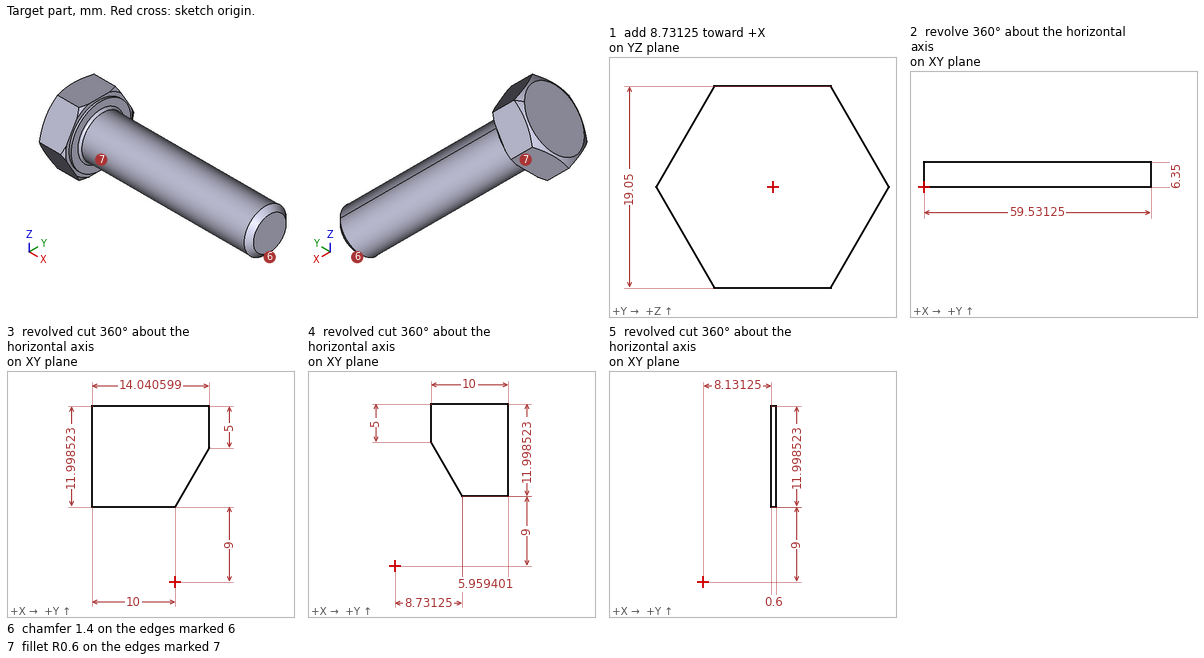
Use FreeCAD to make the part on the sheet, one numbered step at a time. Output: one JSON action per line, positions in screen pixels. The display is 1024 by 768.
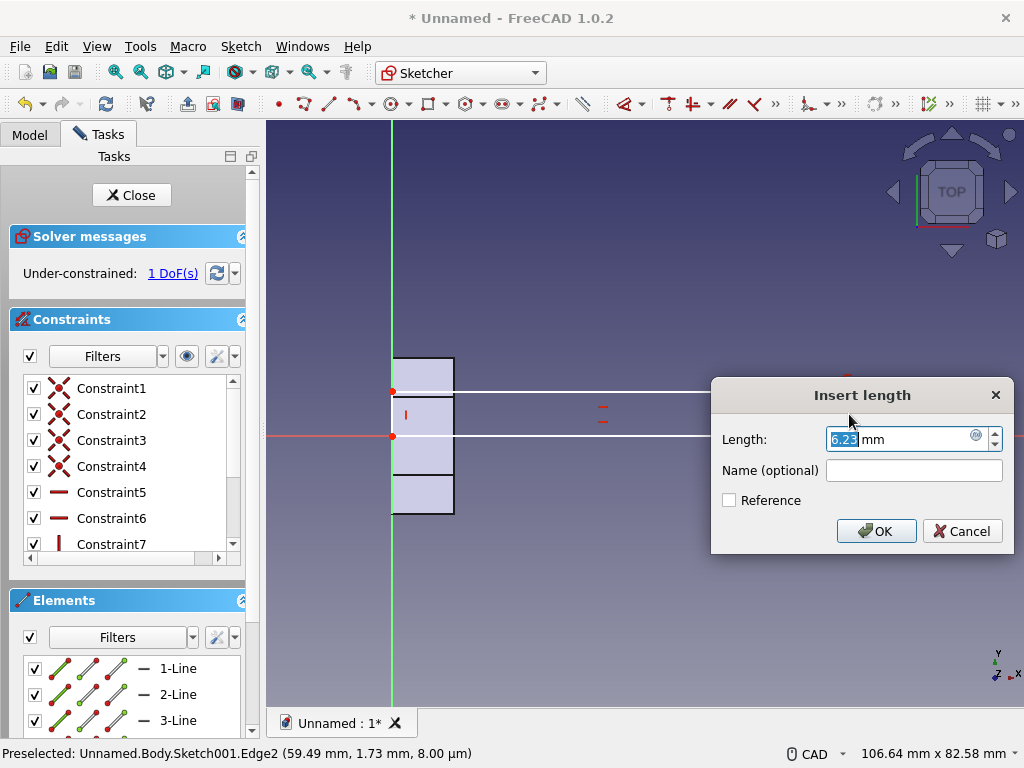
{"action": "type", "text": "6.35"}
{"action": "key", "text": "Return"}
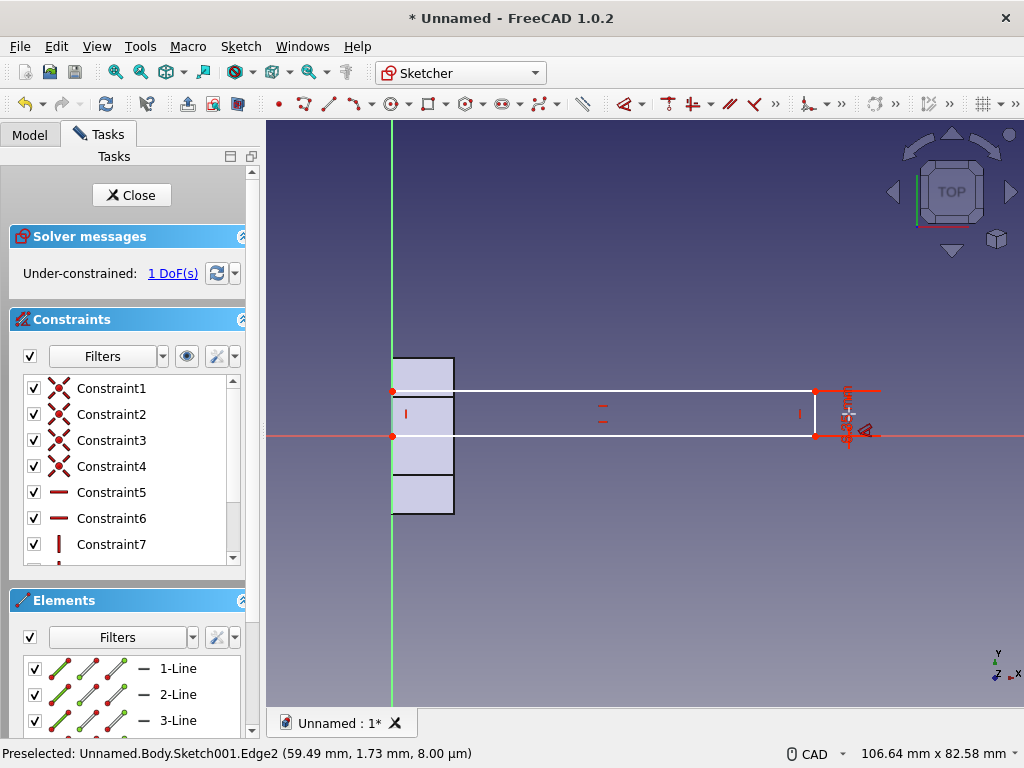
{"action": "left_click", "coordinate": [519, 436]}
{"action": "left_click", "coordinate": [604, 470]}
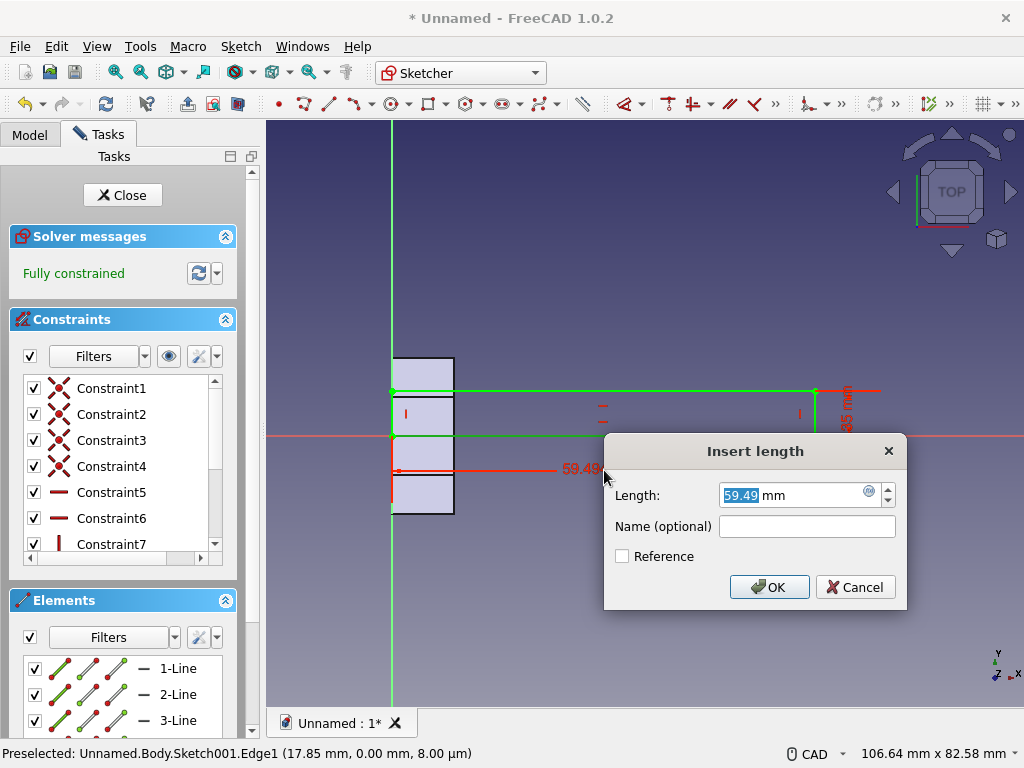
{"action": "type", "text": "59.53125"}
{"action": "key", "text": "Return"}
{"action": "key", "text": "Escape"}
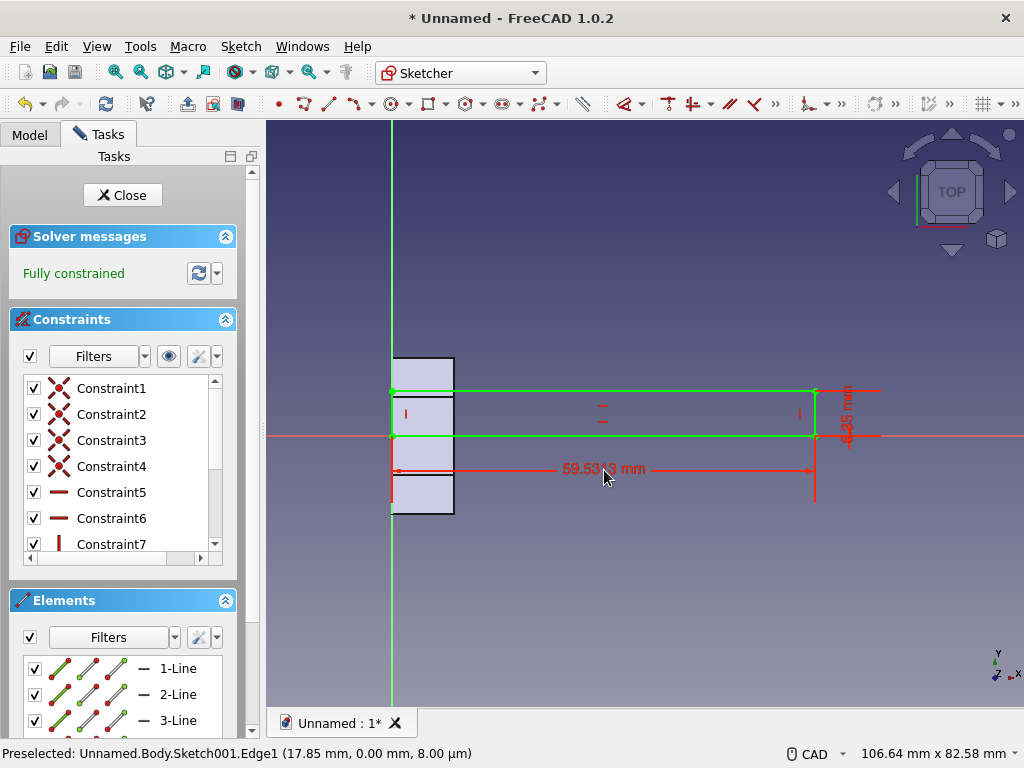
{"action": "left_click", "coordinate": [123, 195]}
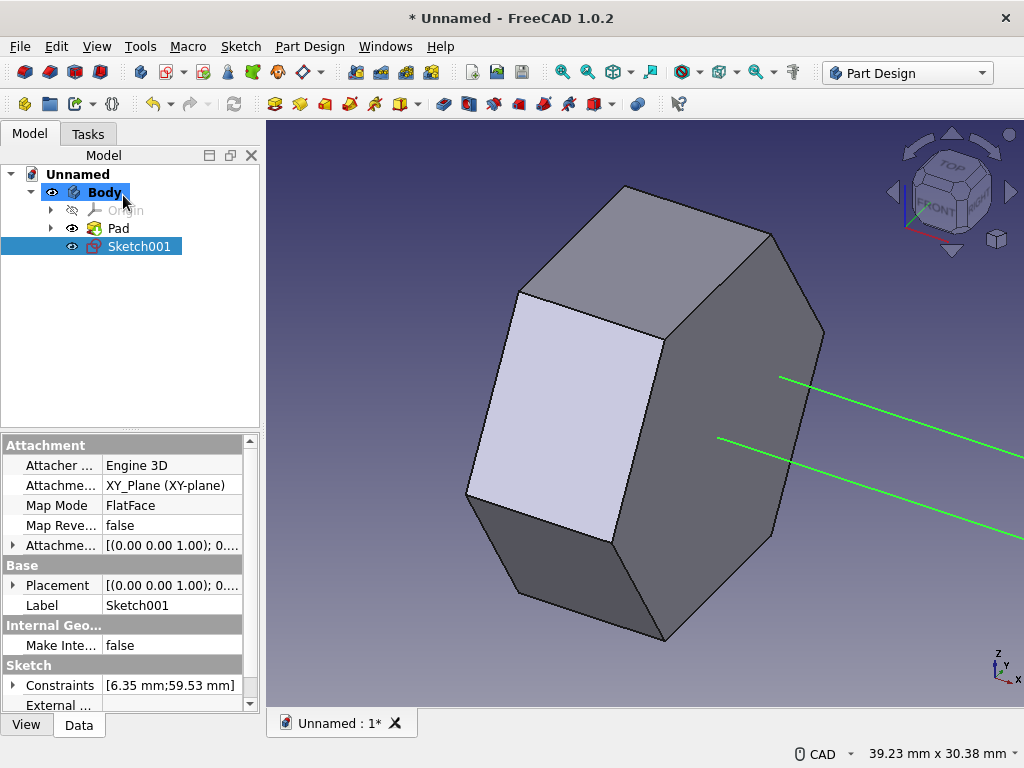
{"action": "left_click", "coordinate": [300, 104]}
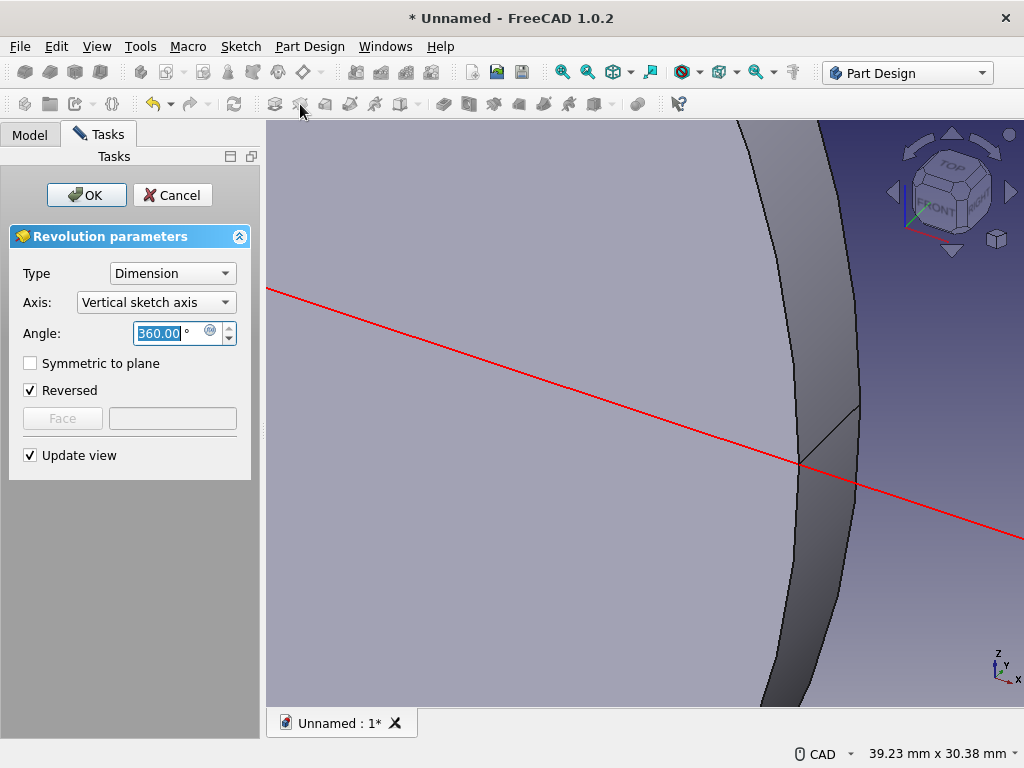
{"action": "left_click", "coordinate": [157, 302]}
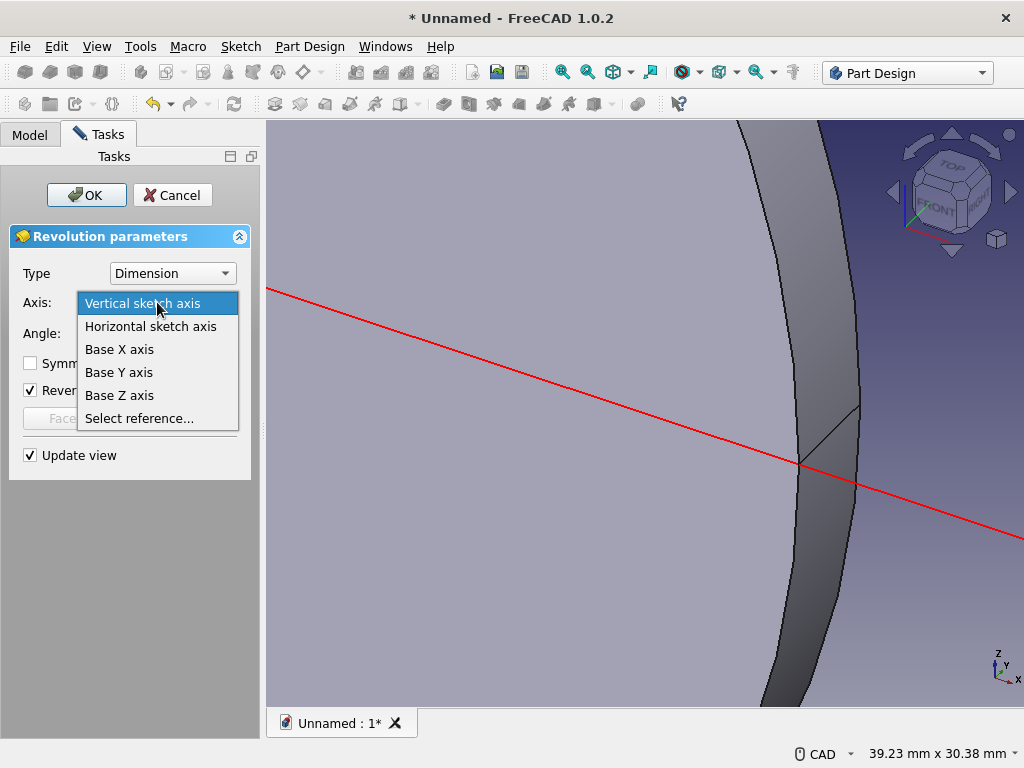
{"action": "left_click", "coordinate": [156, 326]}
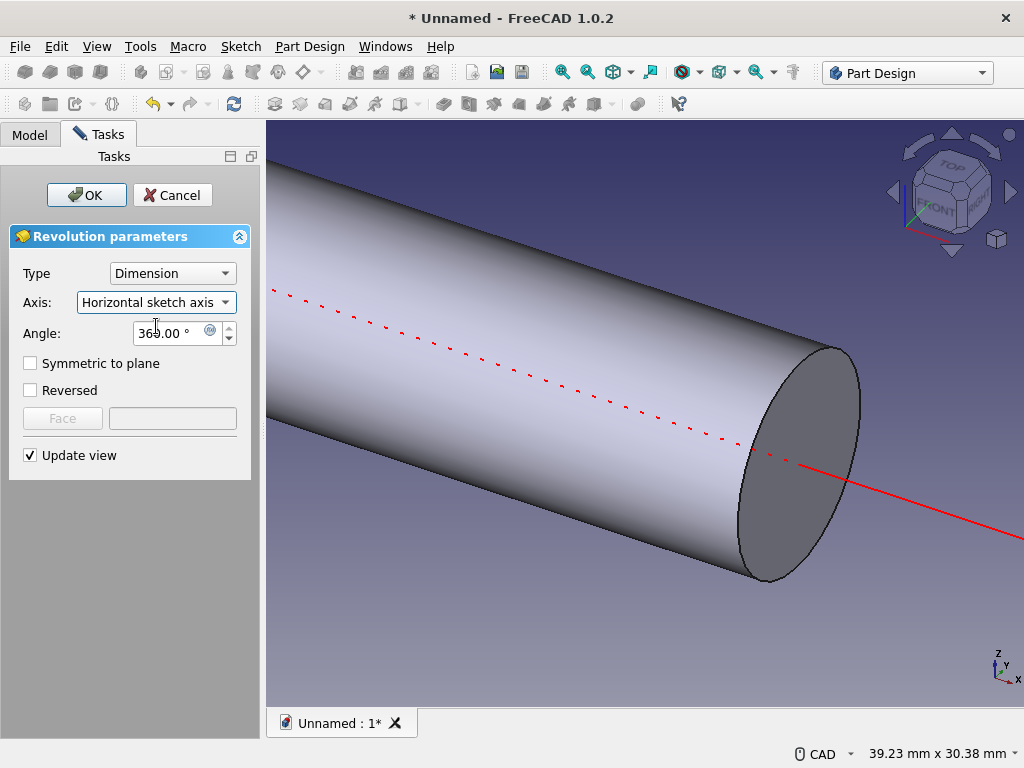
{"action": "left_click", "coordinate": [87, 195]}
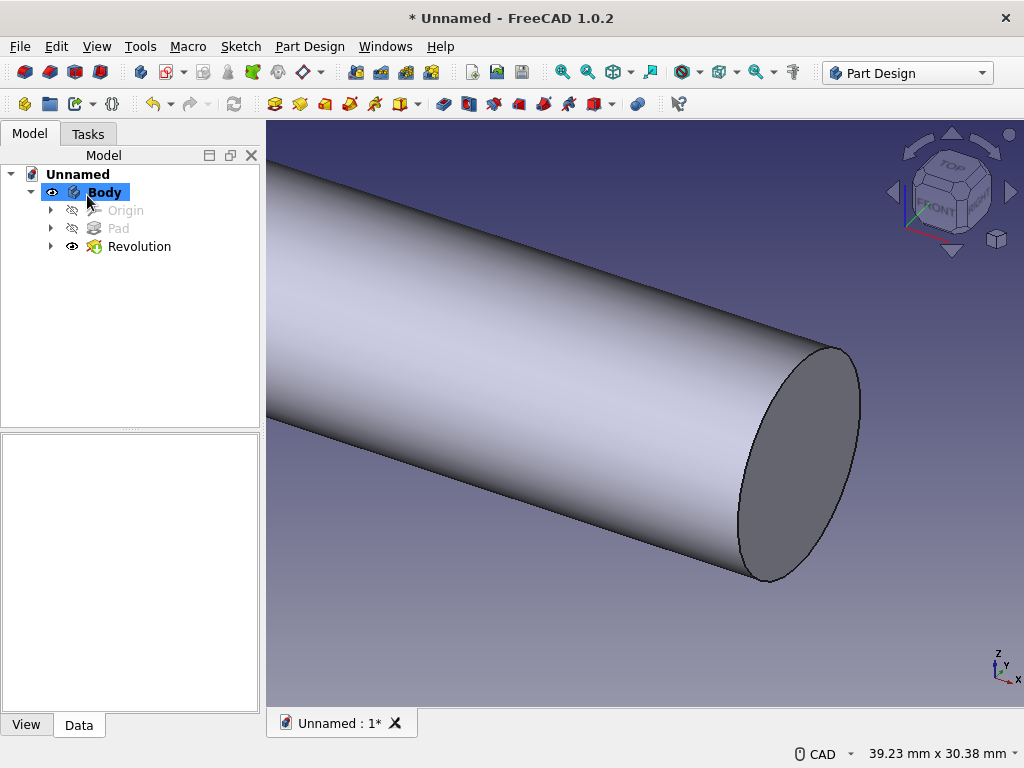
{"action": "left_click", "coordinate": [563, 72]}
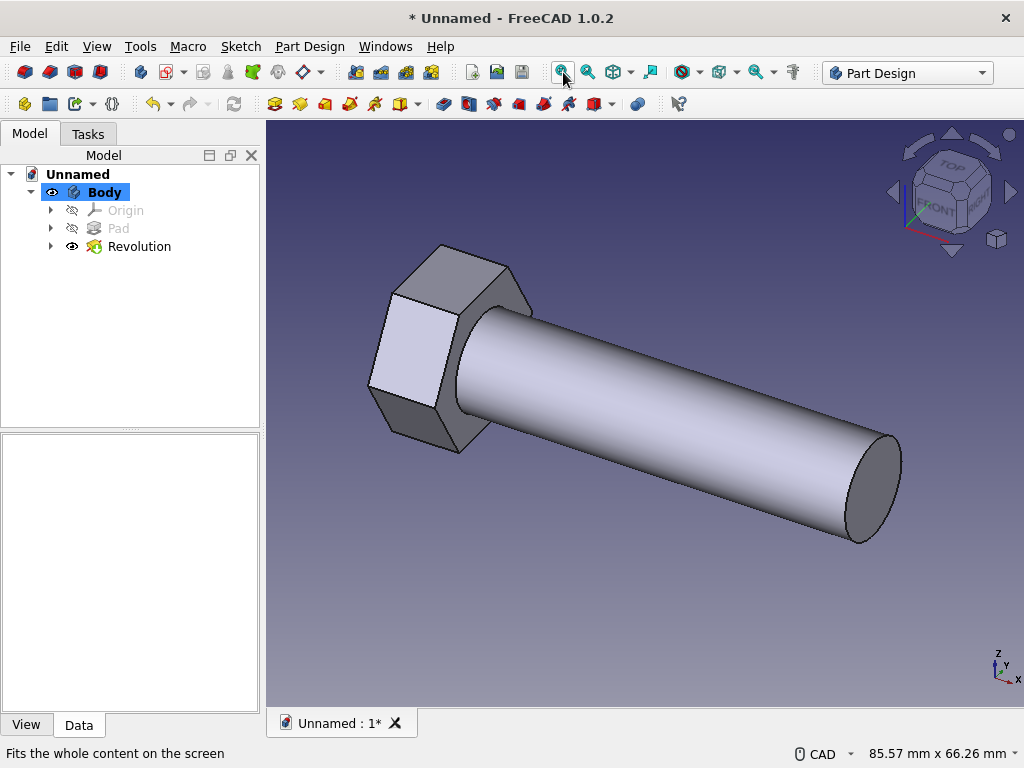
{"action": "left_click", "coordinate": [166, 72]}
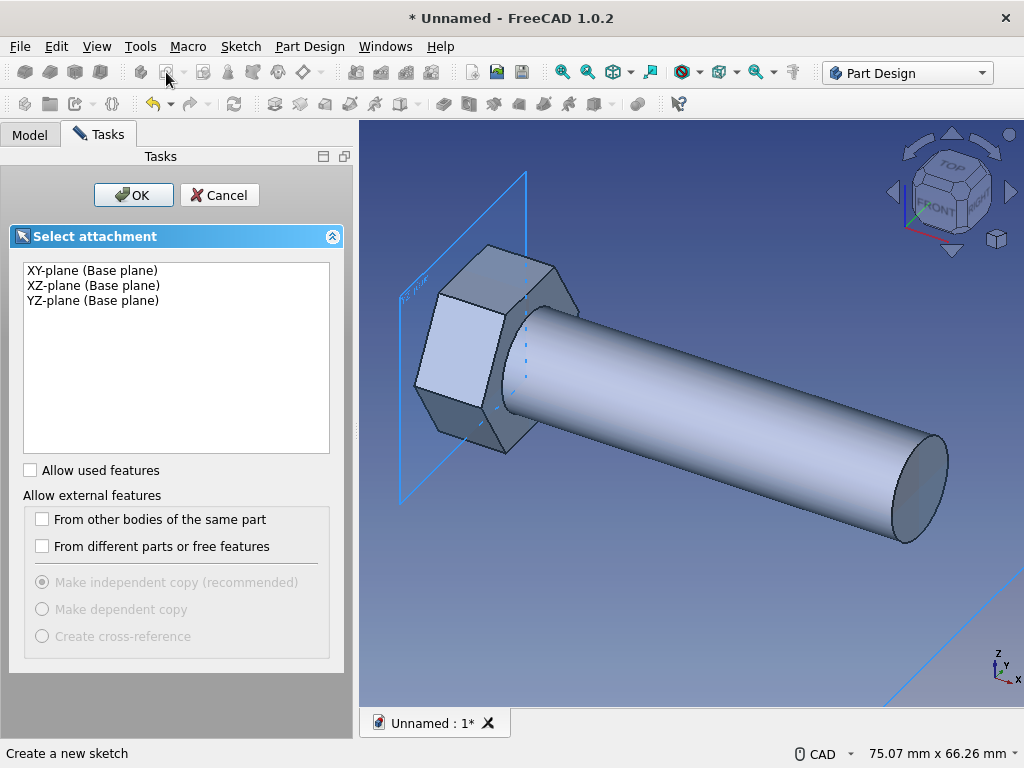
{"action": "left_click", "coordinate": [84, 270]}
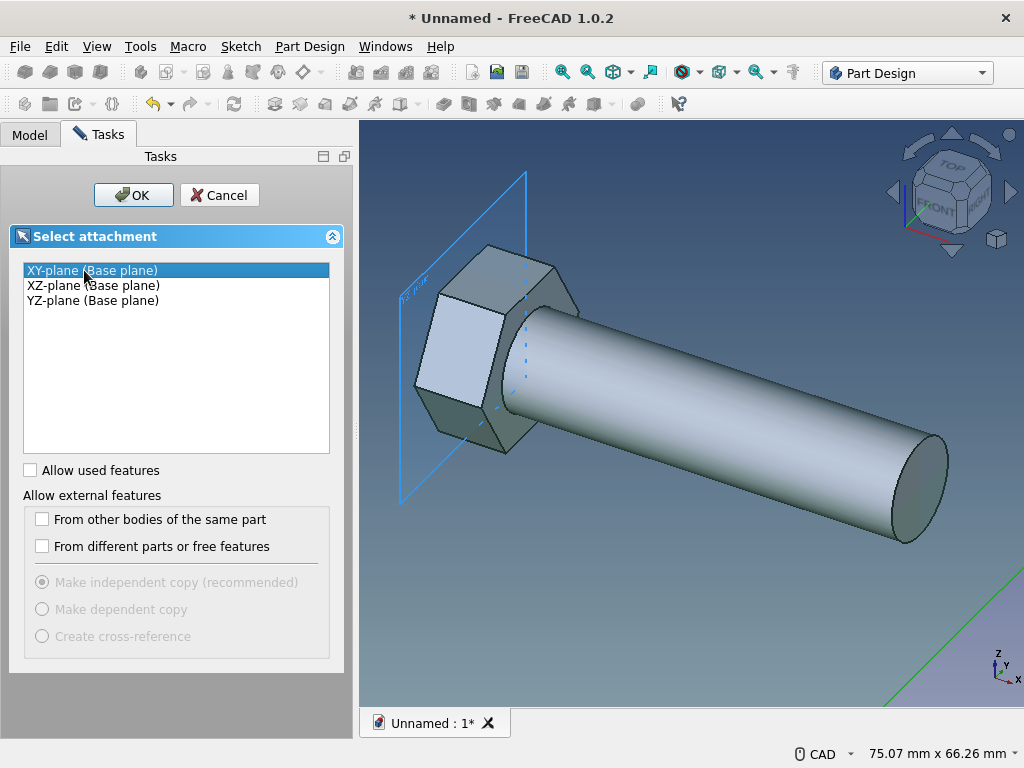
{"action": "left_click", "coordinate": [134, 195]}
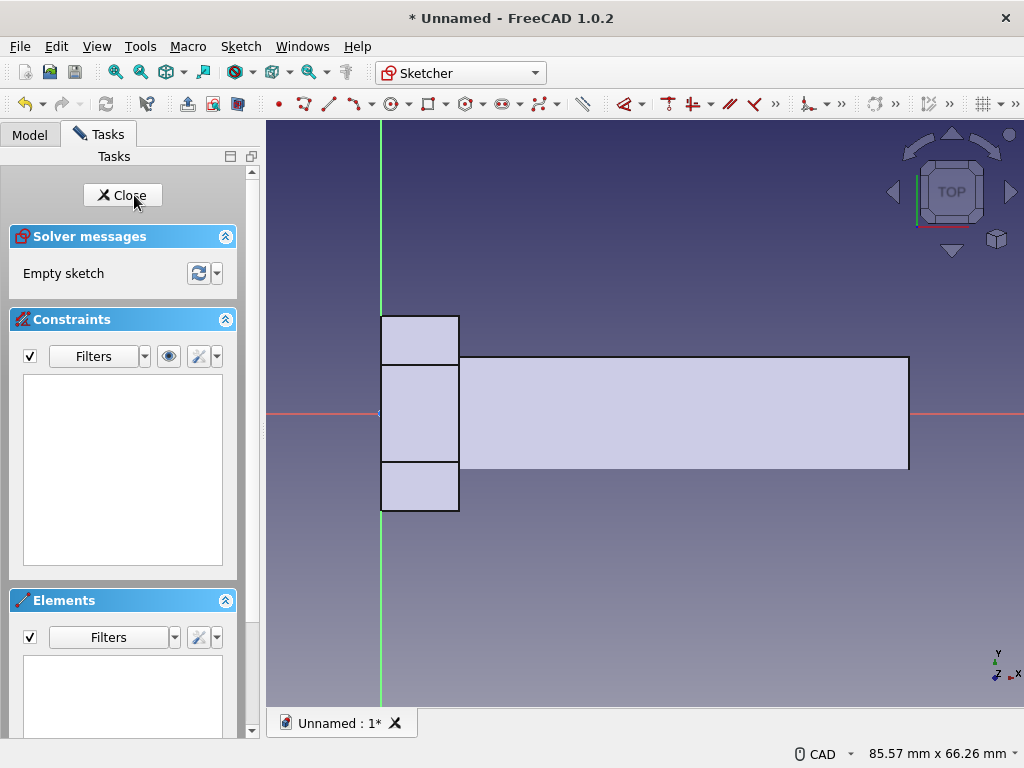
{"action": "left_click", "coordinate": [238, 104]}